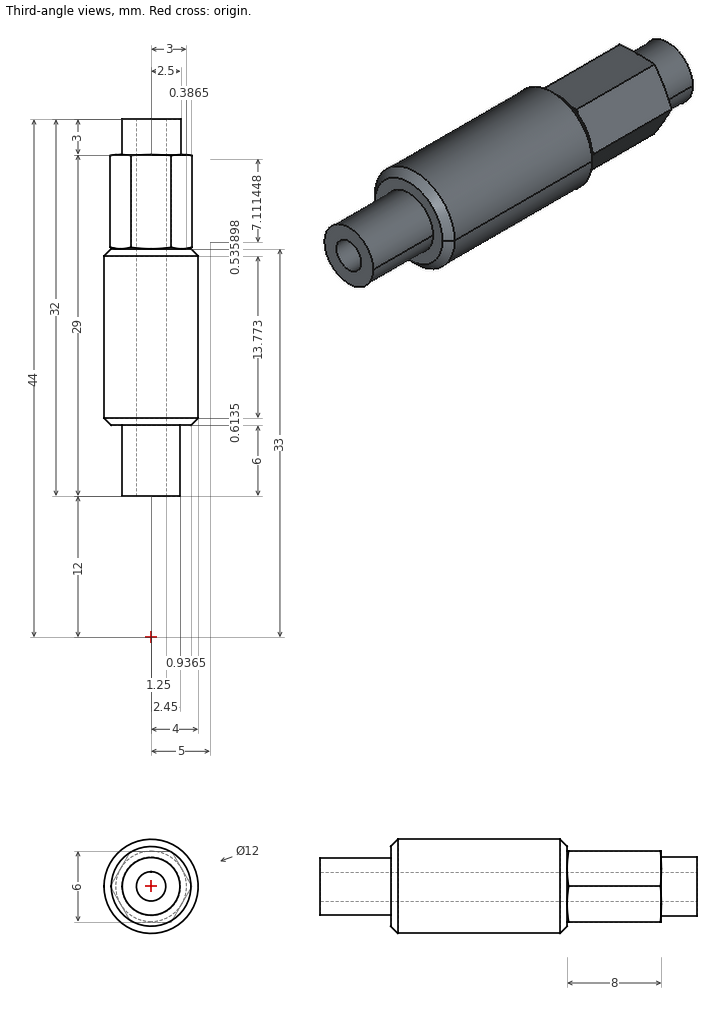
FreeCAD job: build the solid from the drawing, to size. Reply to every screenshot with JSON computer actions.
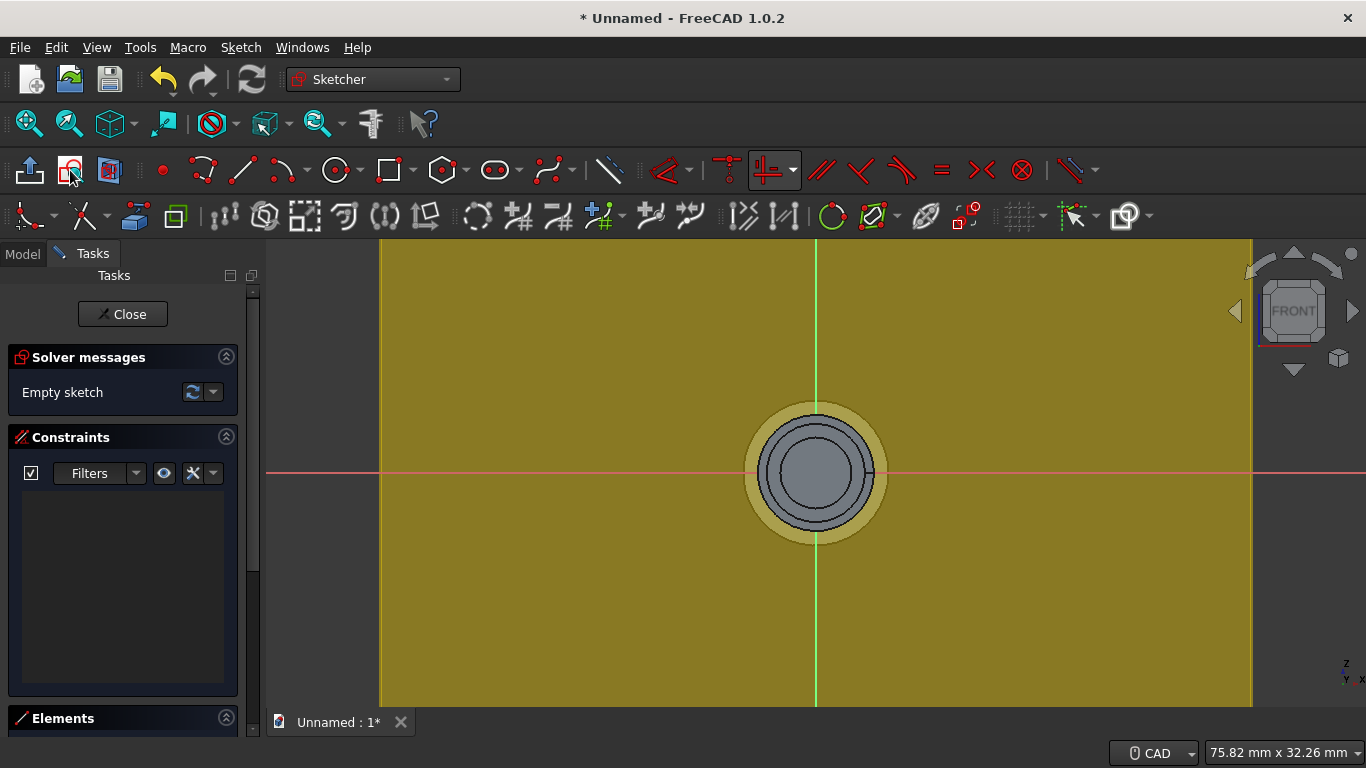
{"action": "left_click", "coordinate": [110, 170]}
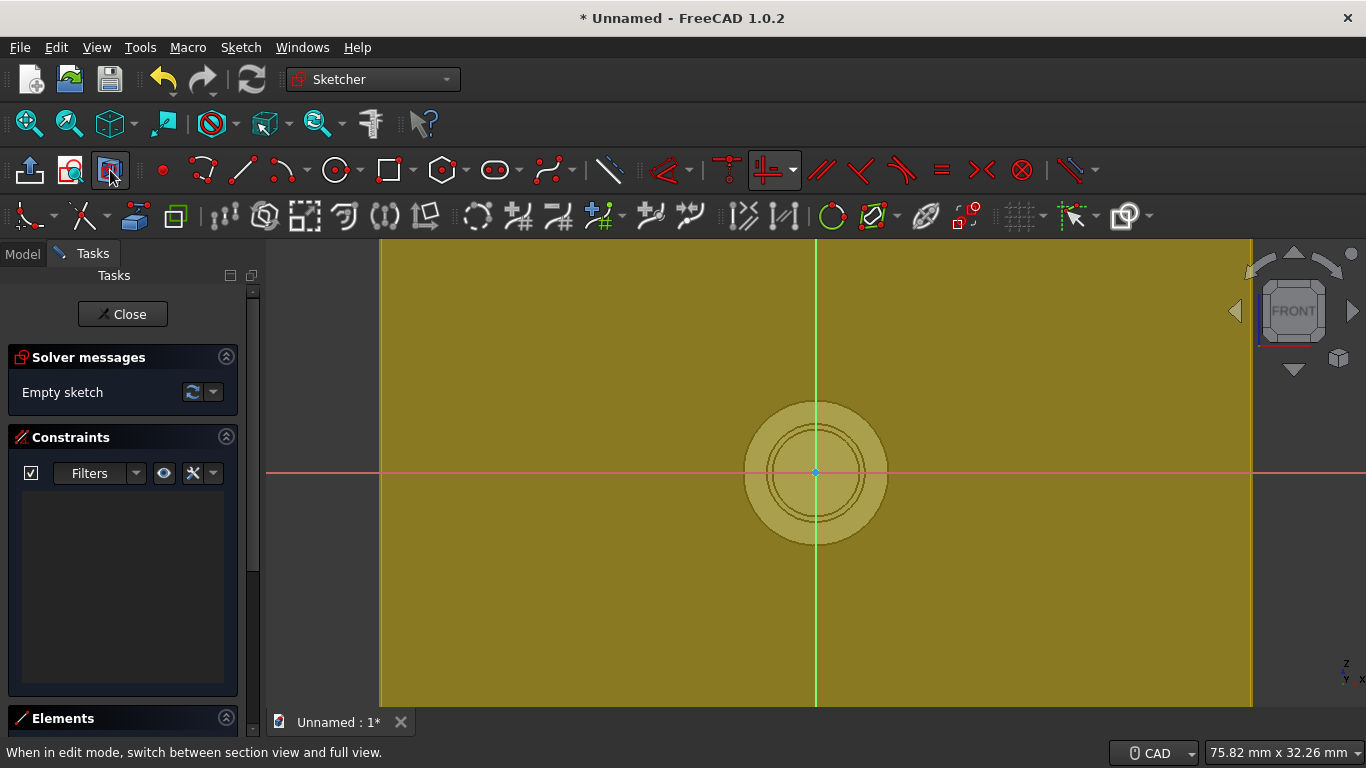
{"action": "scroll", "coordinate": [899, 473], "scroll_direction": "up", "scroll_amount": 3}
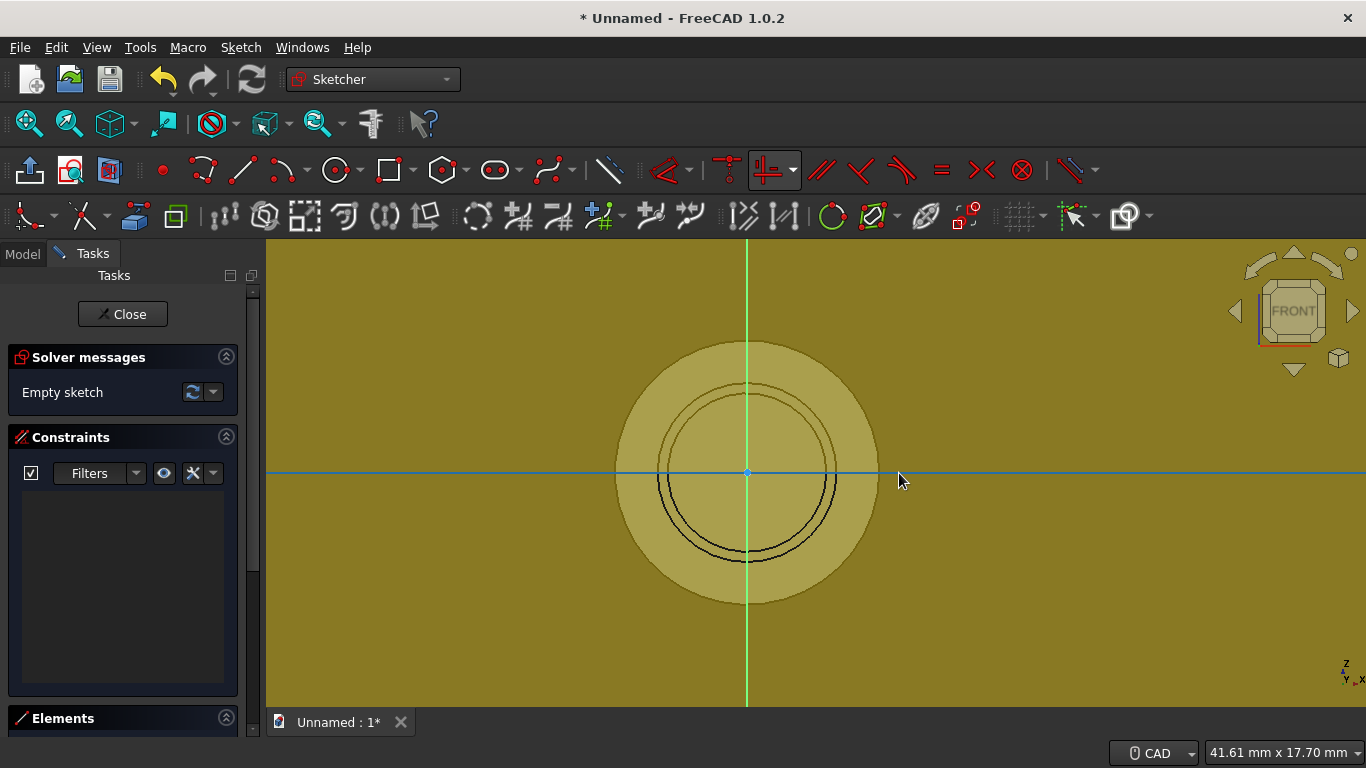
{"action": "left_click", "coordinate": [442, 170]}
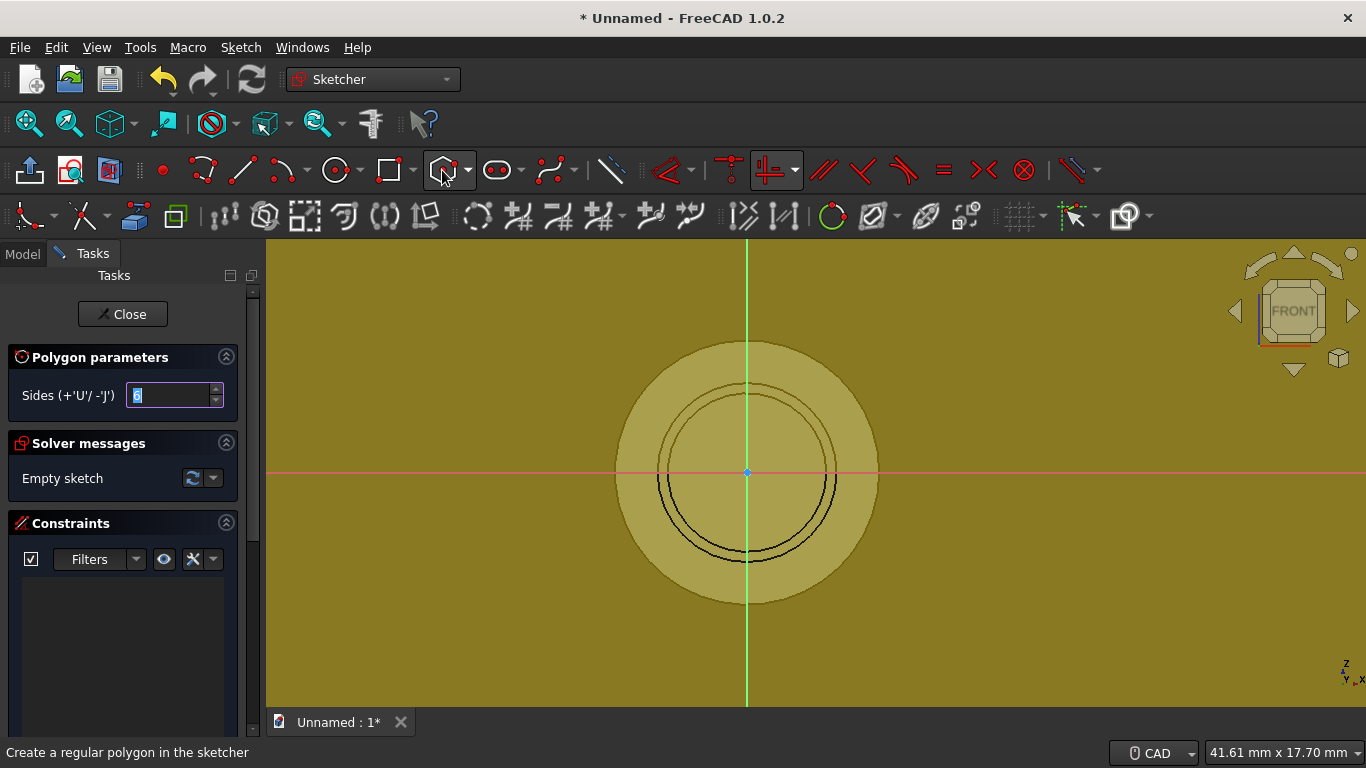
{"action": "left_click", "coordinate": [747, 473]}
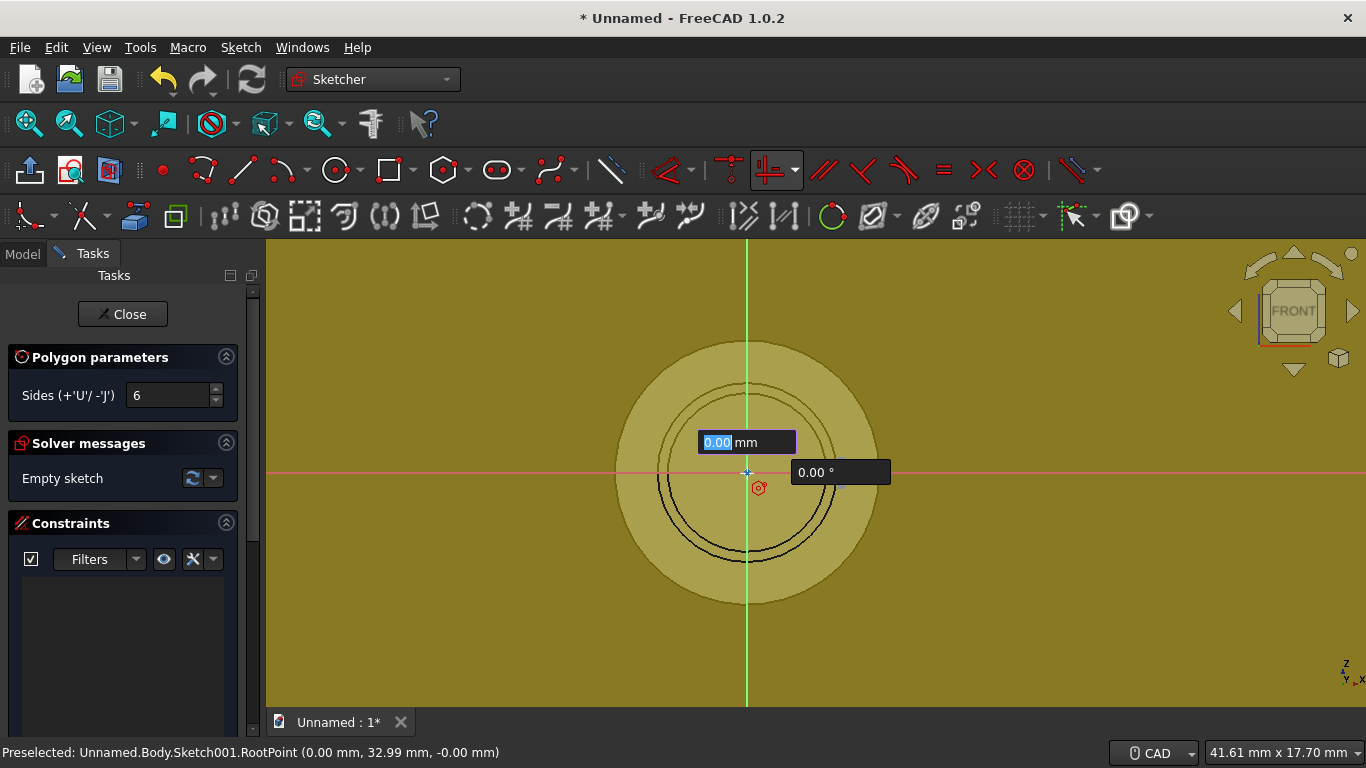
{"action": "left_click", "coordinate": [655, 473]}
{"action": "right_click", "coordinate": [655, 473]}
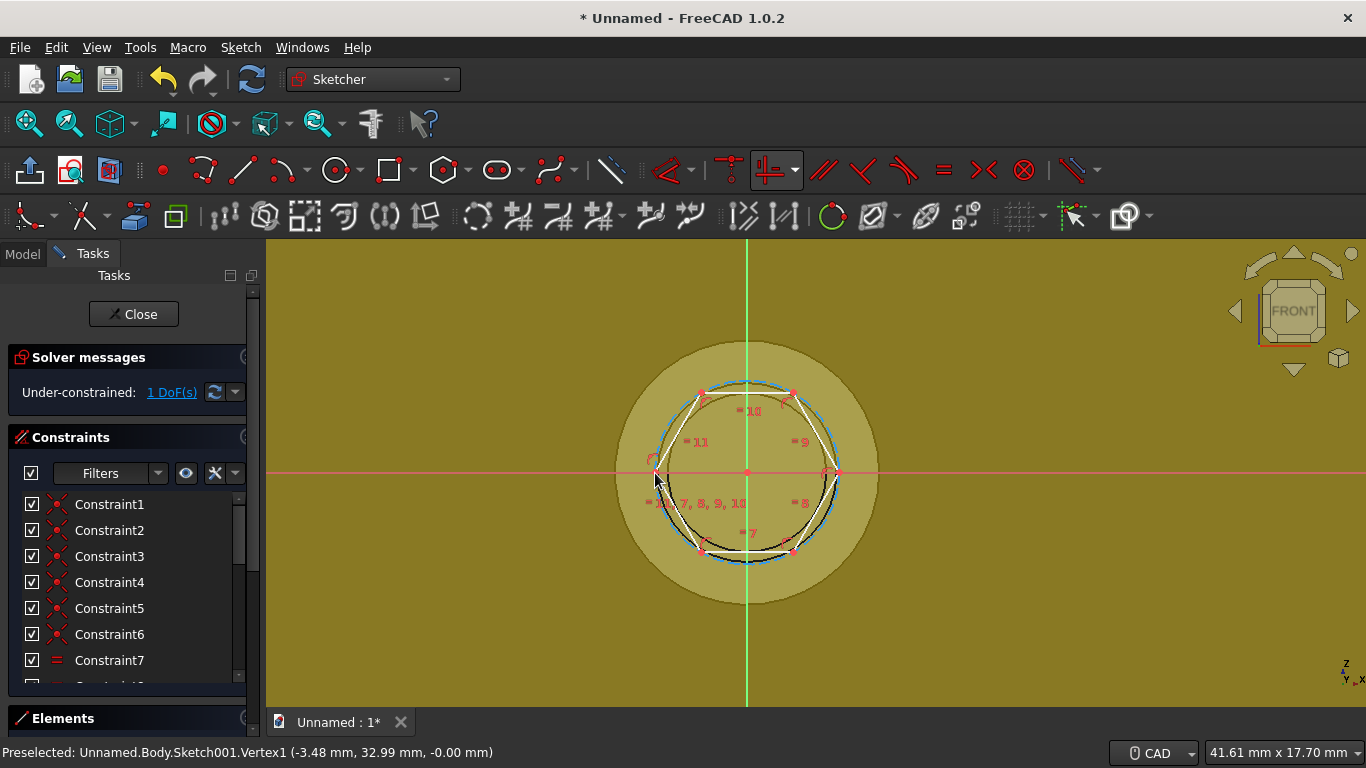
{"action": "left_click", "coordinate": [336, 170]}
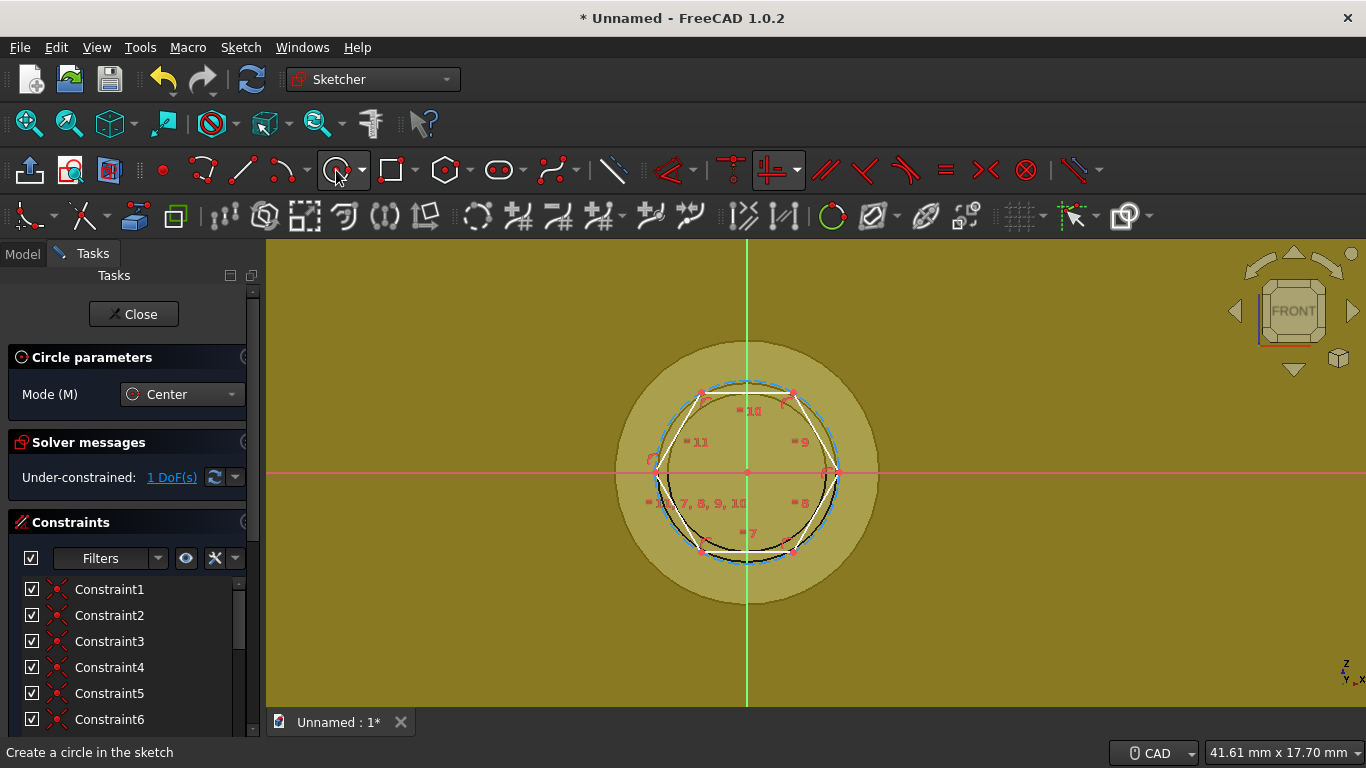
{"action": "left_click", "coordinate": [747, 473]}
{"action": "left_click", "coordinate": [859, 360]}
{"action": "key", "text": "Escape"}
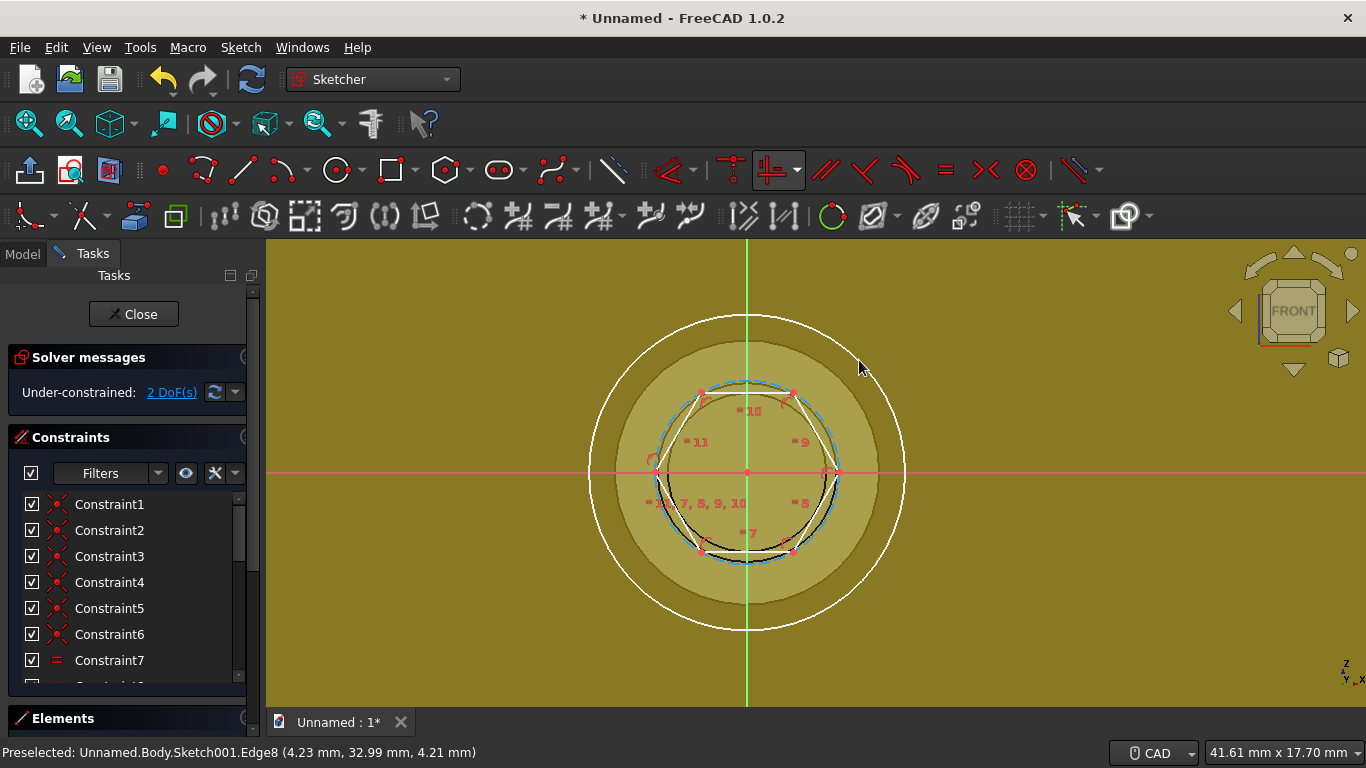
{"action": "left_click", "coordinate": [668, 170]}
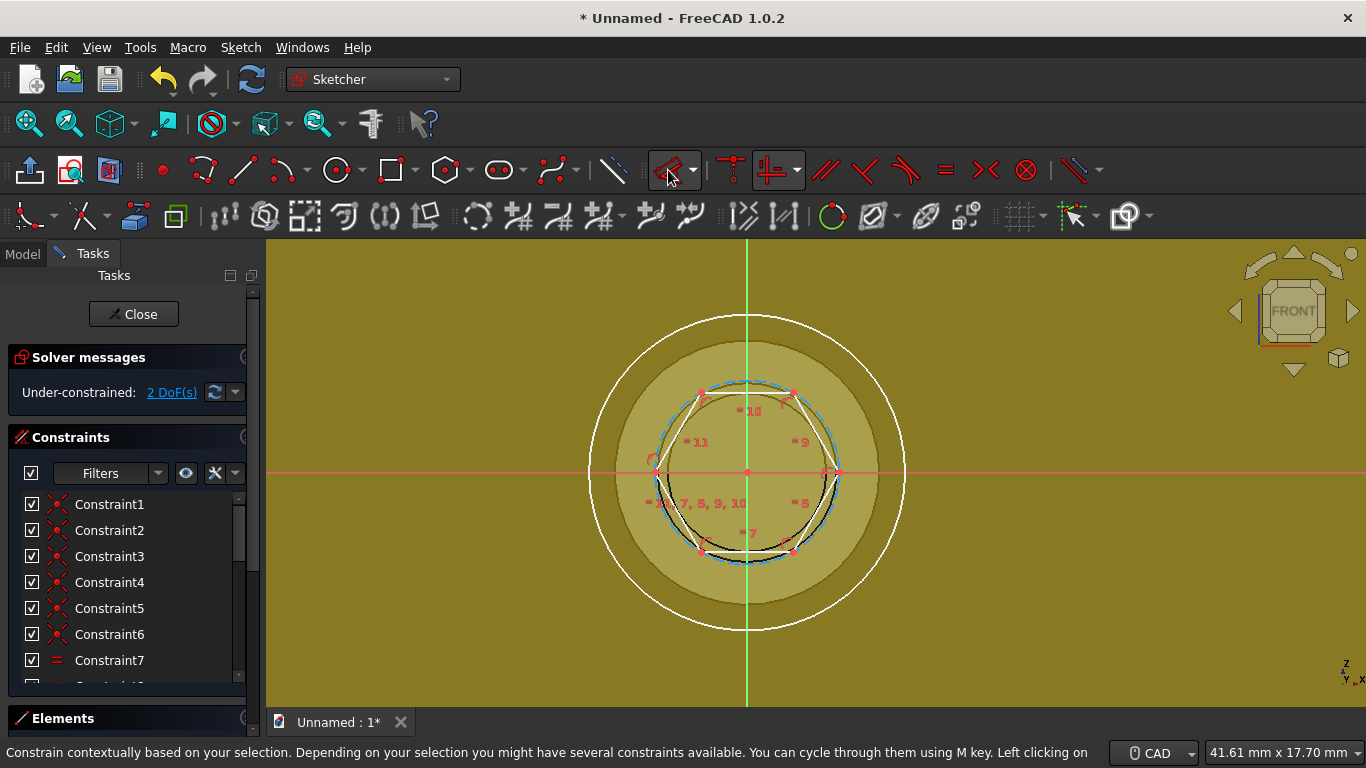
{"action": "left_click", "coordinate": [858, 360]}
{"action": "left_click", "coordinate": [880, 337]}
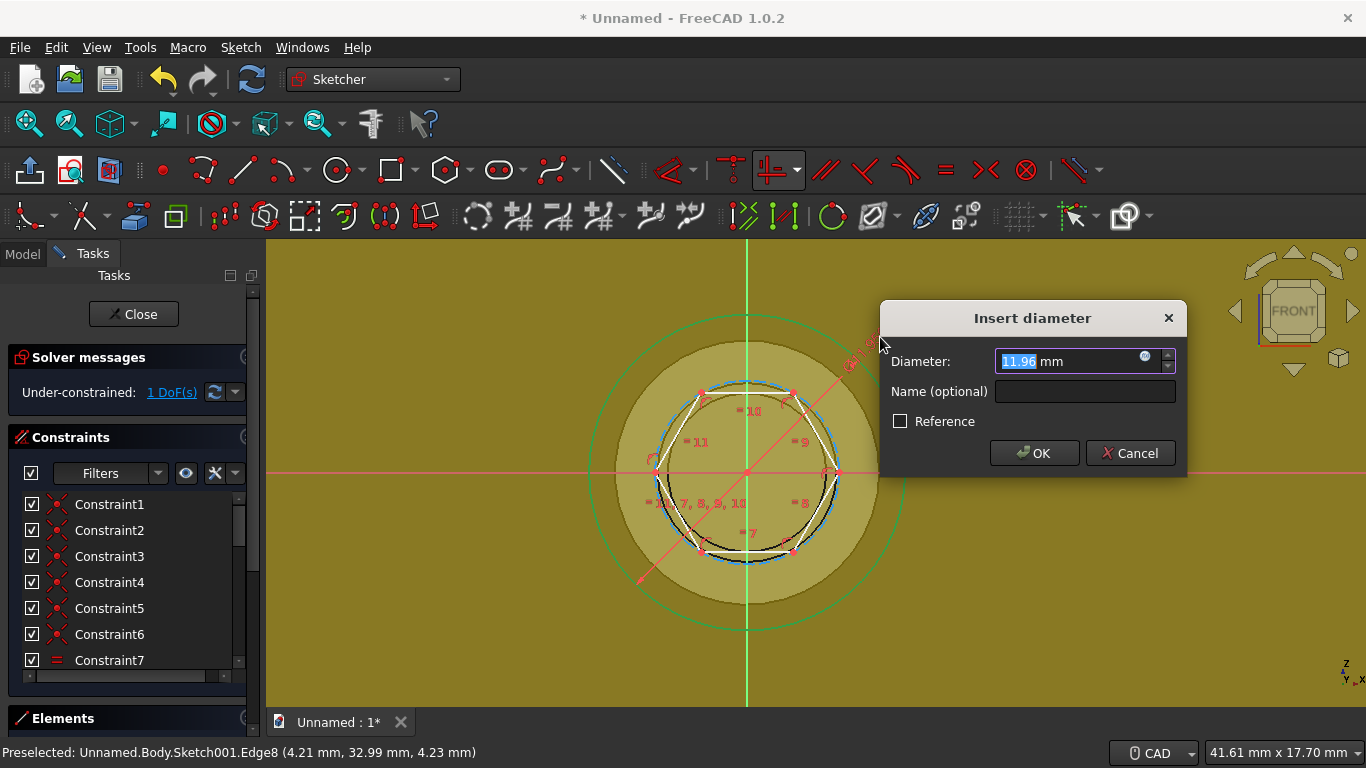
{"action": "type", "text": "12"}
{"action": "key", "text": "Return"}